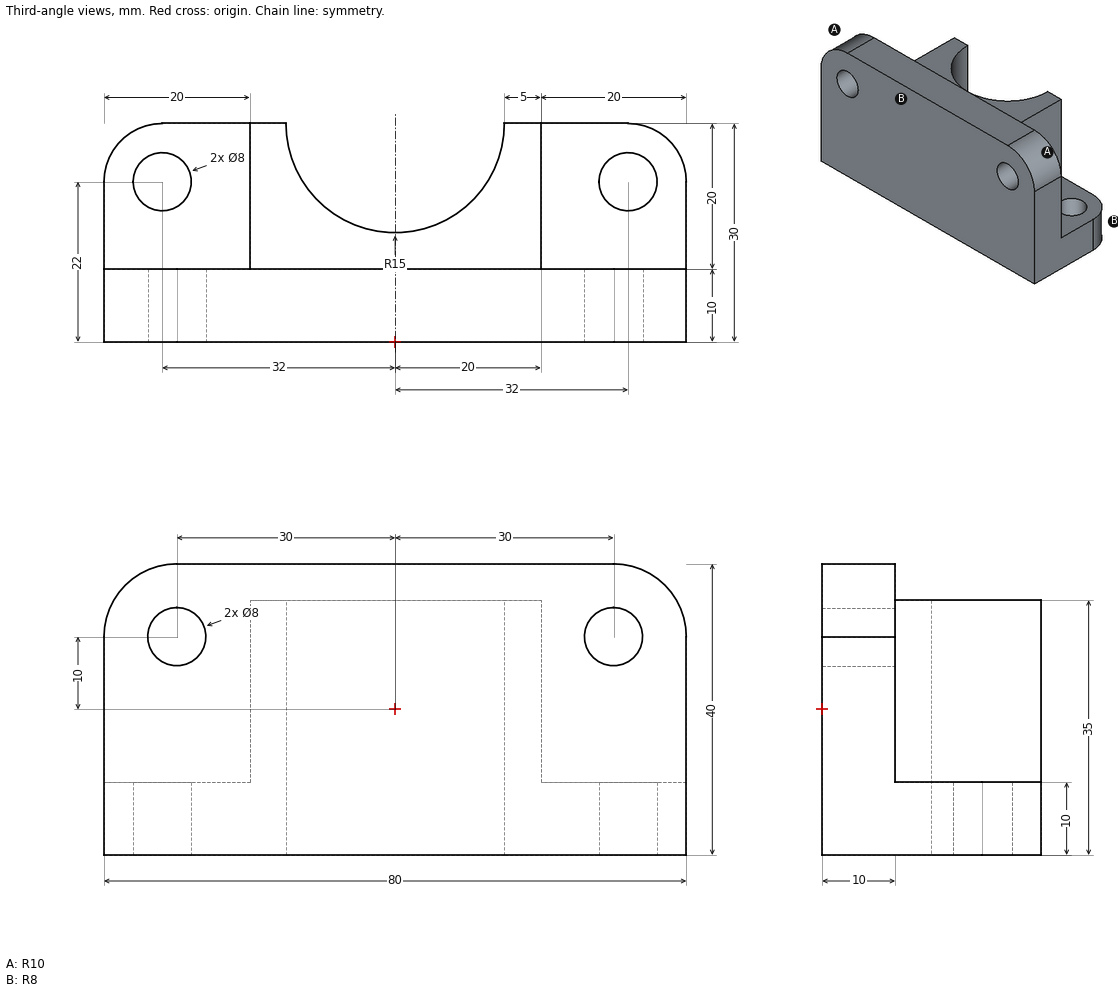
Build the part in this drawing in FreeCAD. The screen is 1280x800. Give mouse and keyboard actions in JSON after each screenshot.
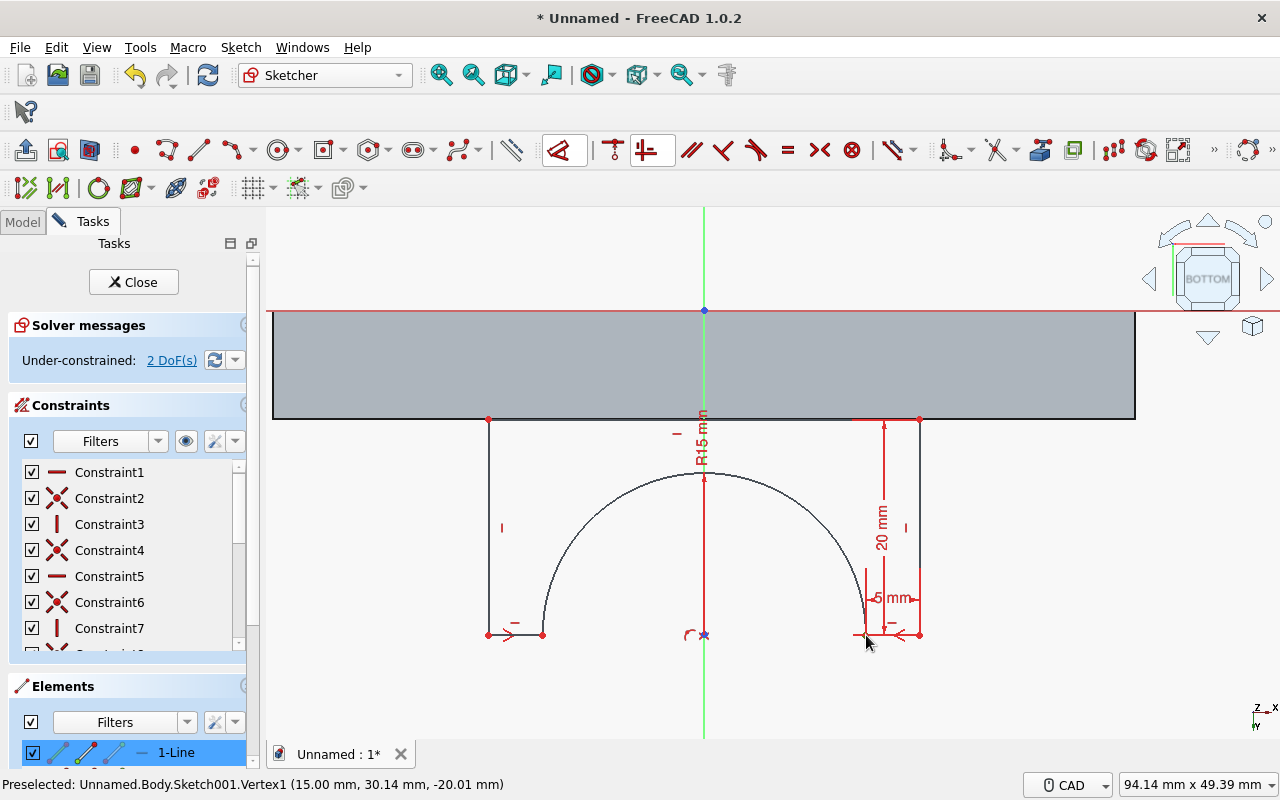
{"action": "key", "text": "i"}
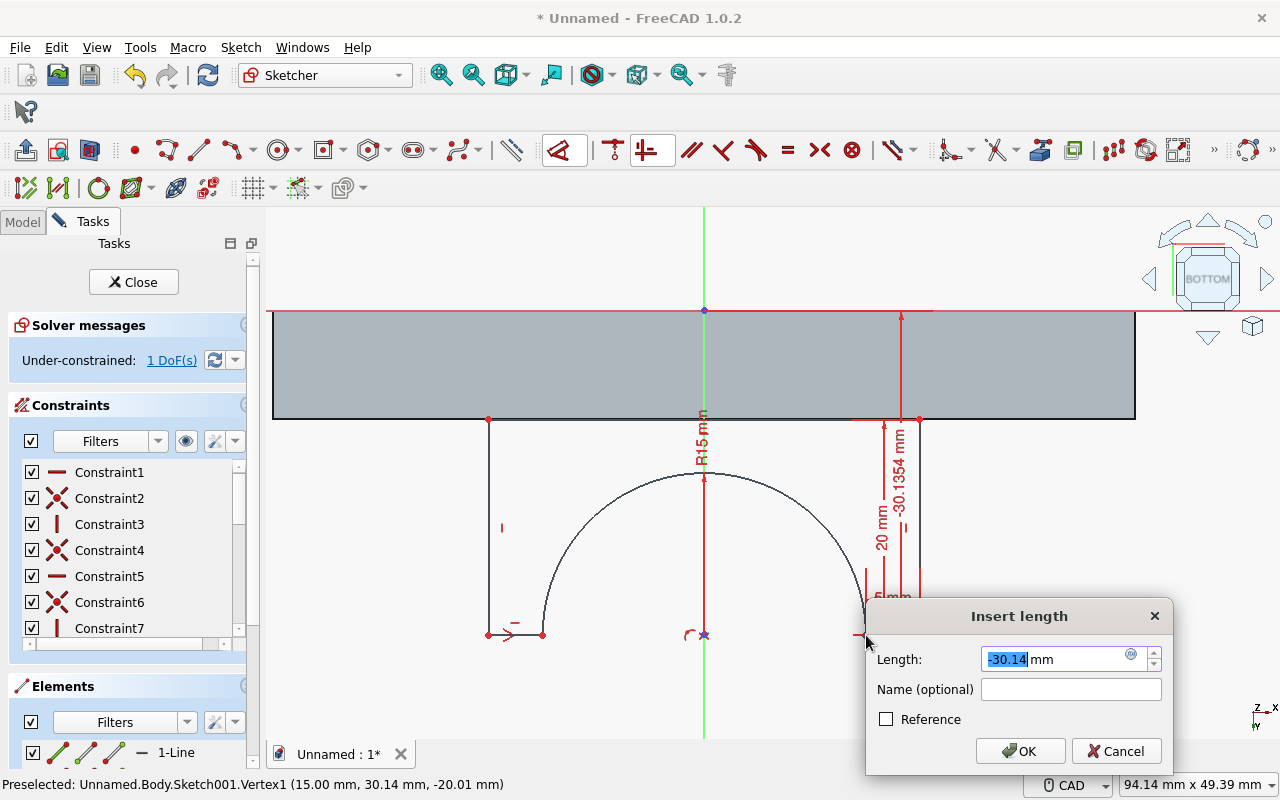
{"action": "type", "text": "-30"}
{"action": "key", "text": "Return"}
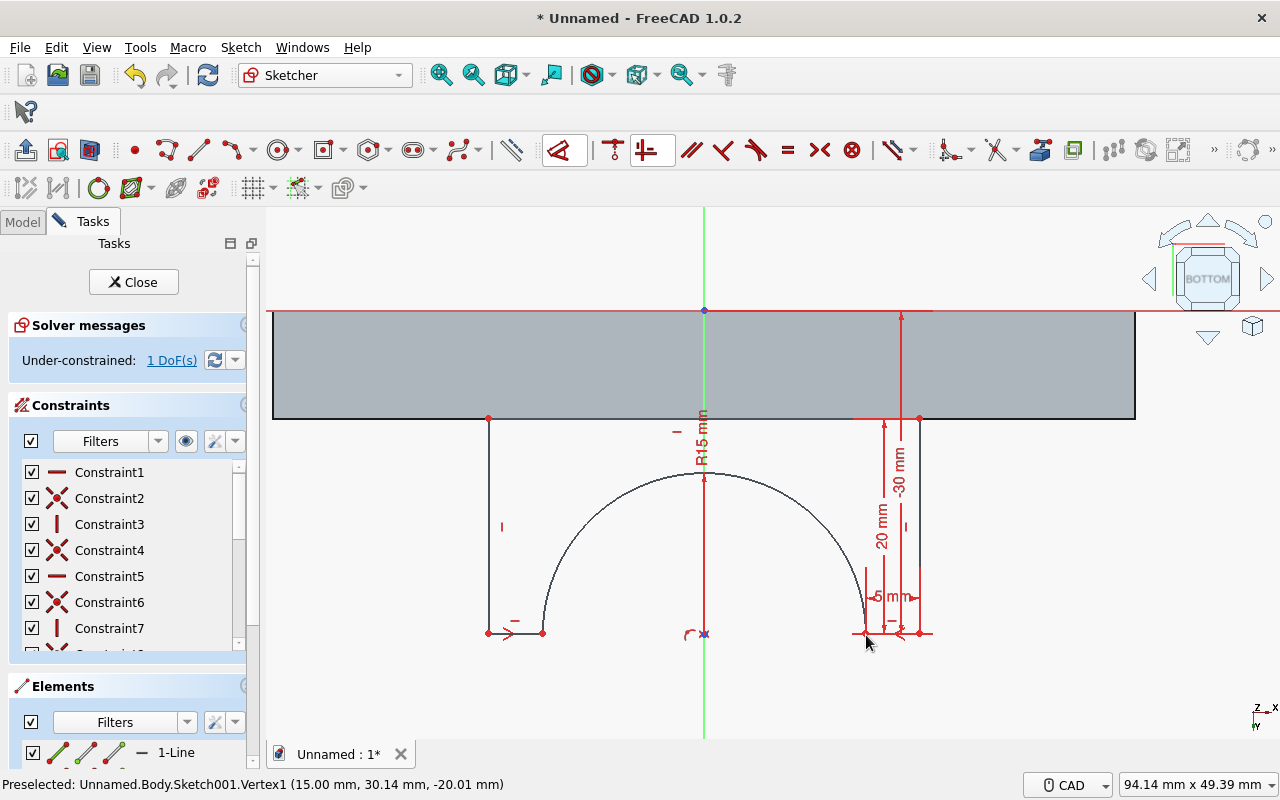
{"action": "left_click", "coordinate": [704, 635]}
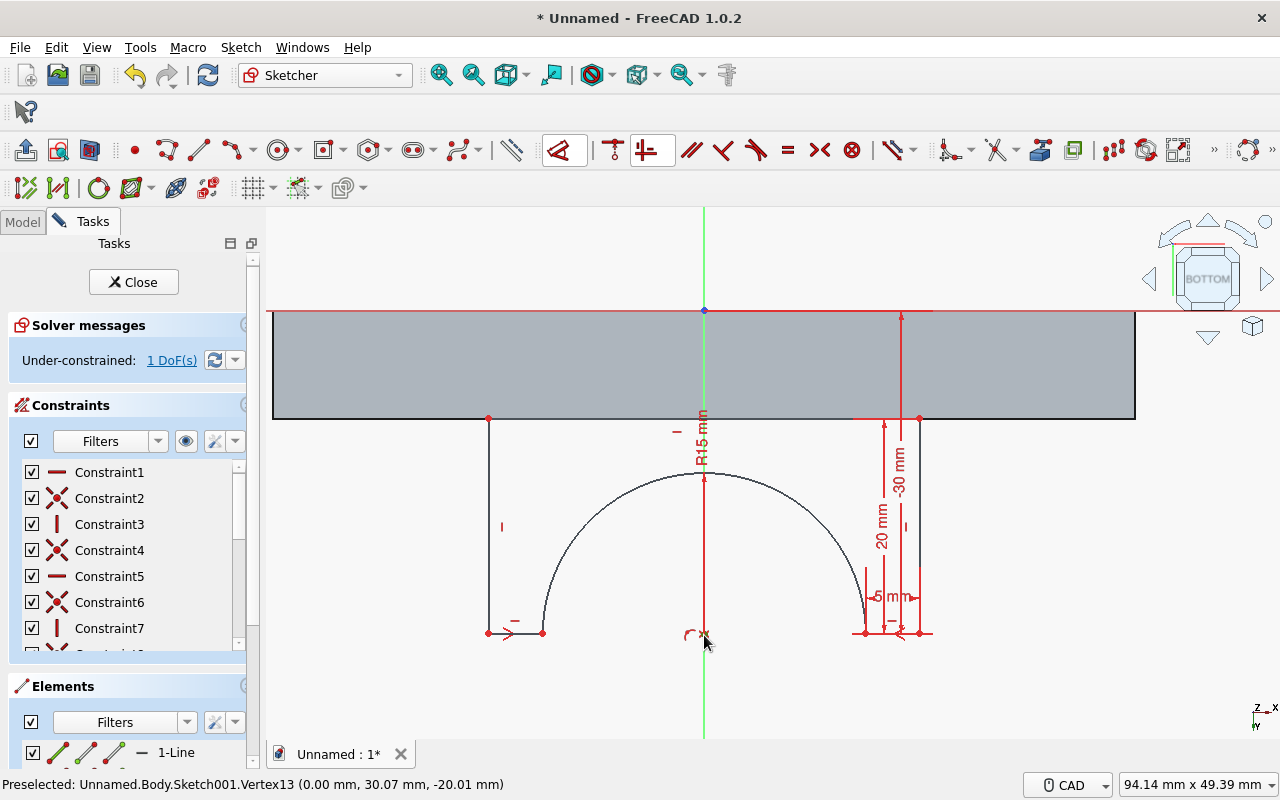
{"action": "left_click", "coordinate": [582, 150]}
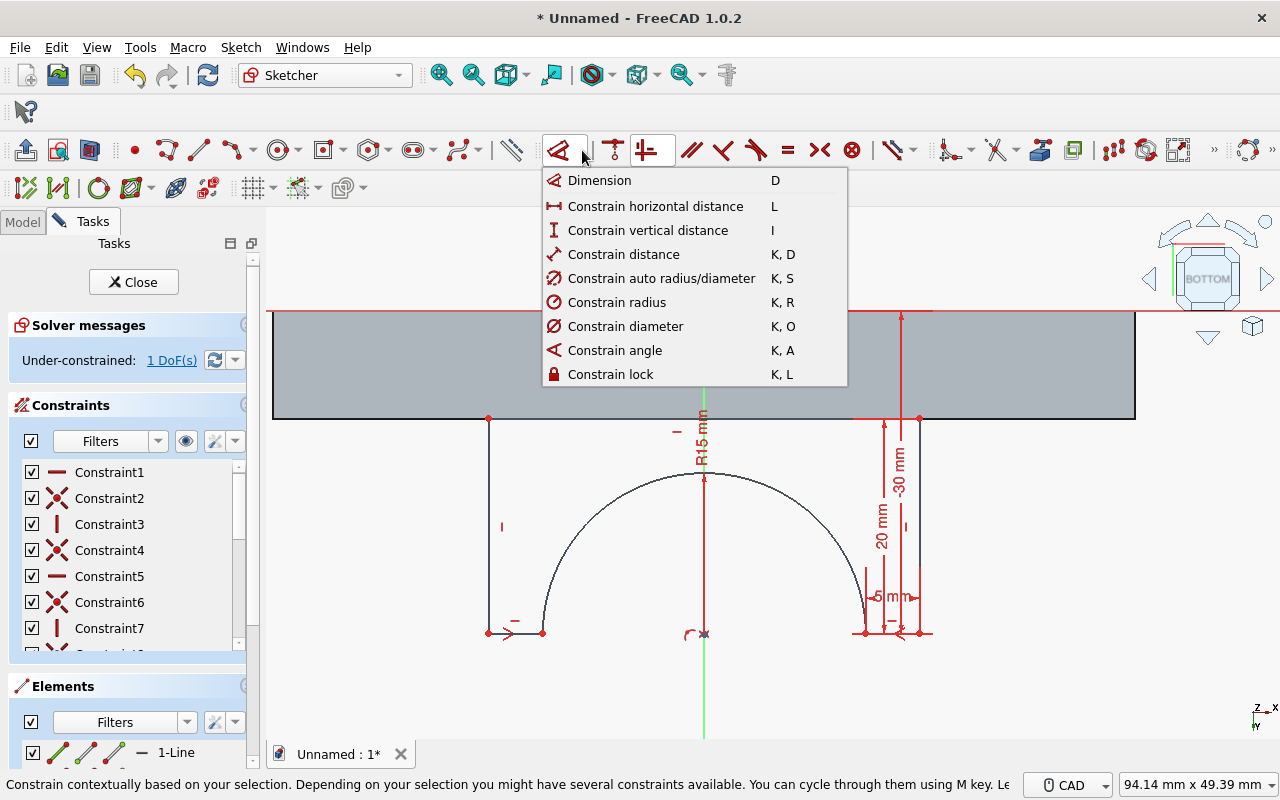
{"action": "left_click", "coordinate": [695, 230]}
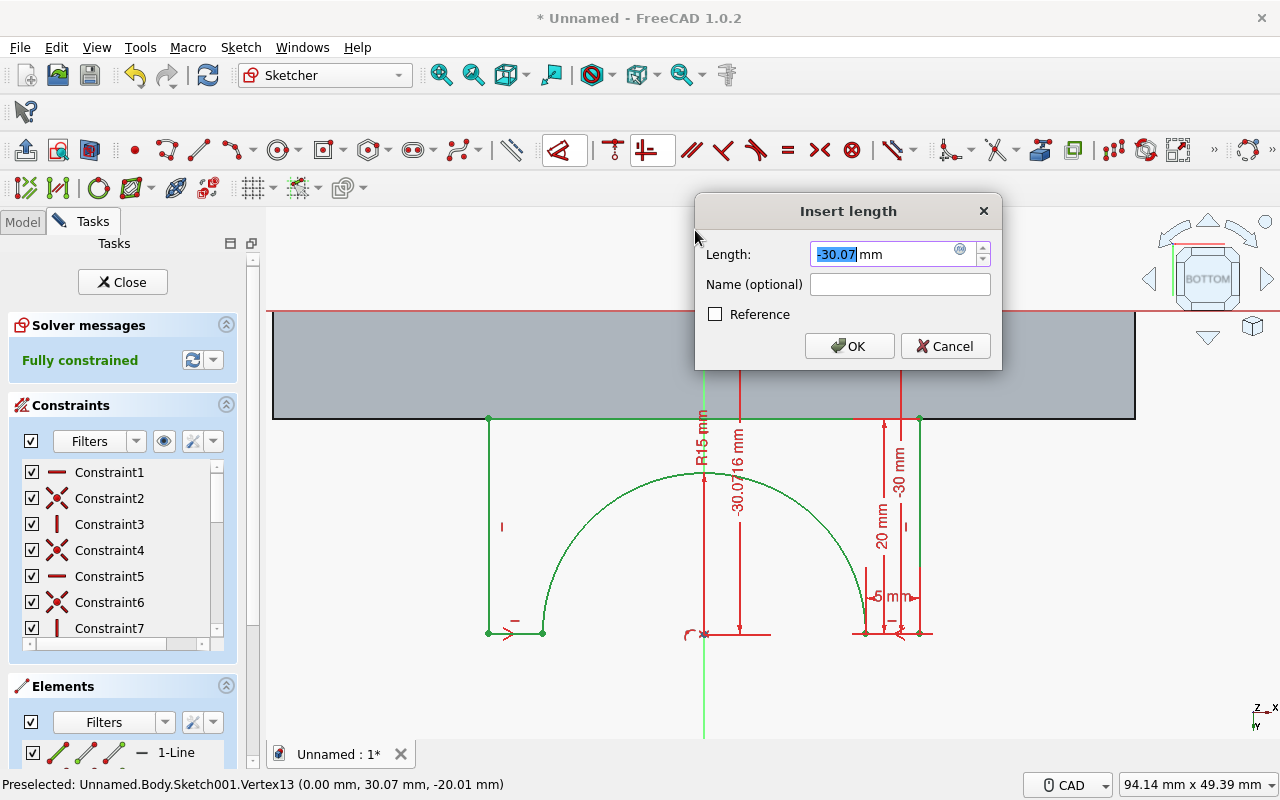
{"action": "type", "text": "-30"}
{"action": "key", "text": "Return"}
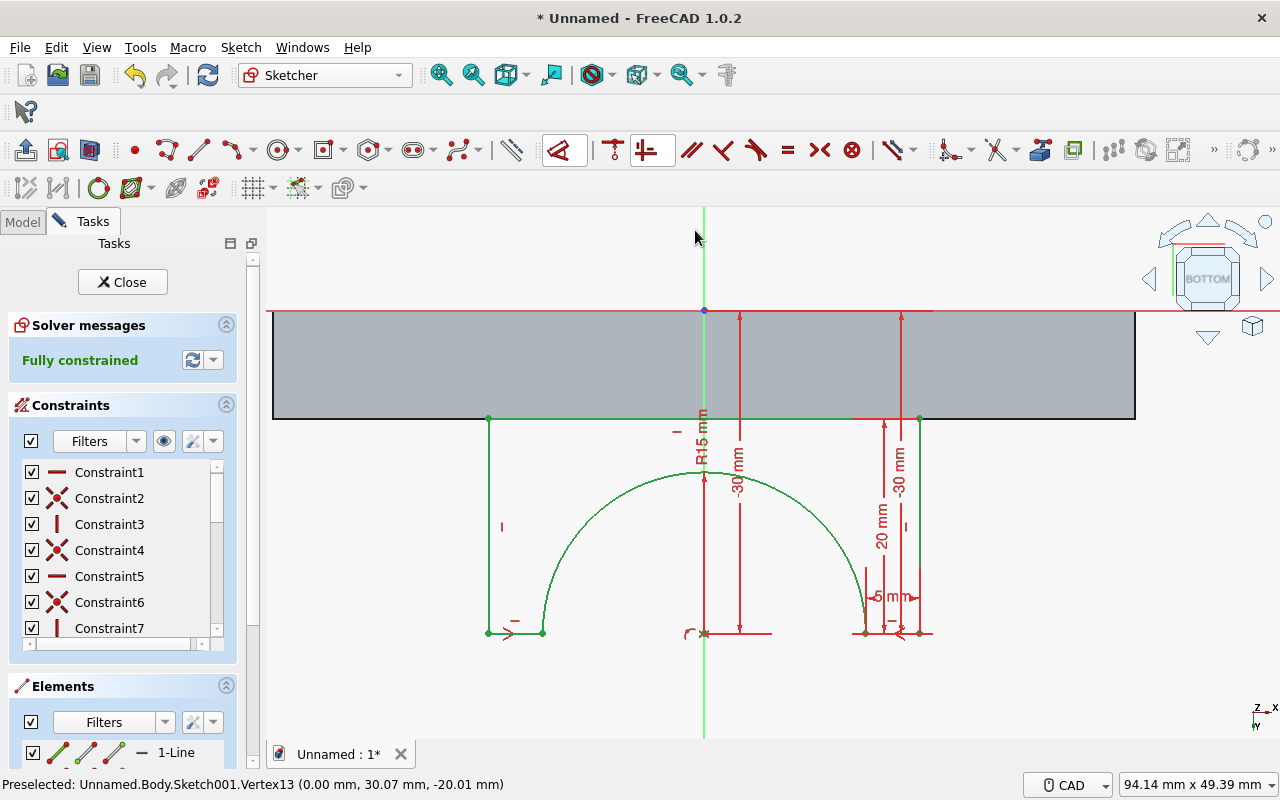
{"action": "left_click", "coordinate": [123, 282]}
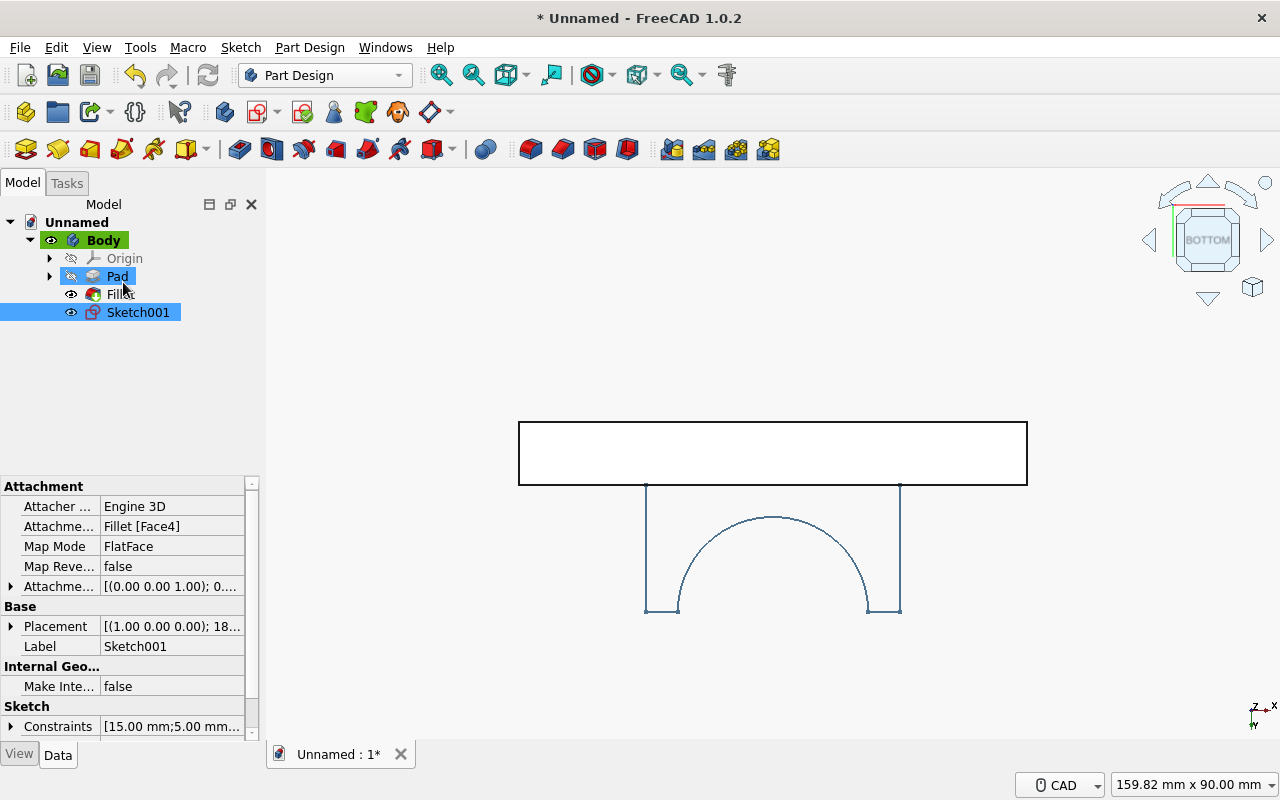
{"action": "left_click", "coordinate": [26, 150]}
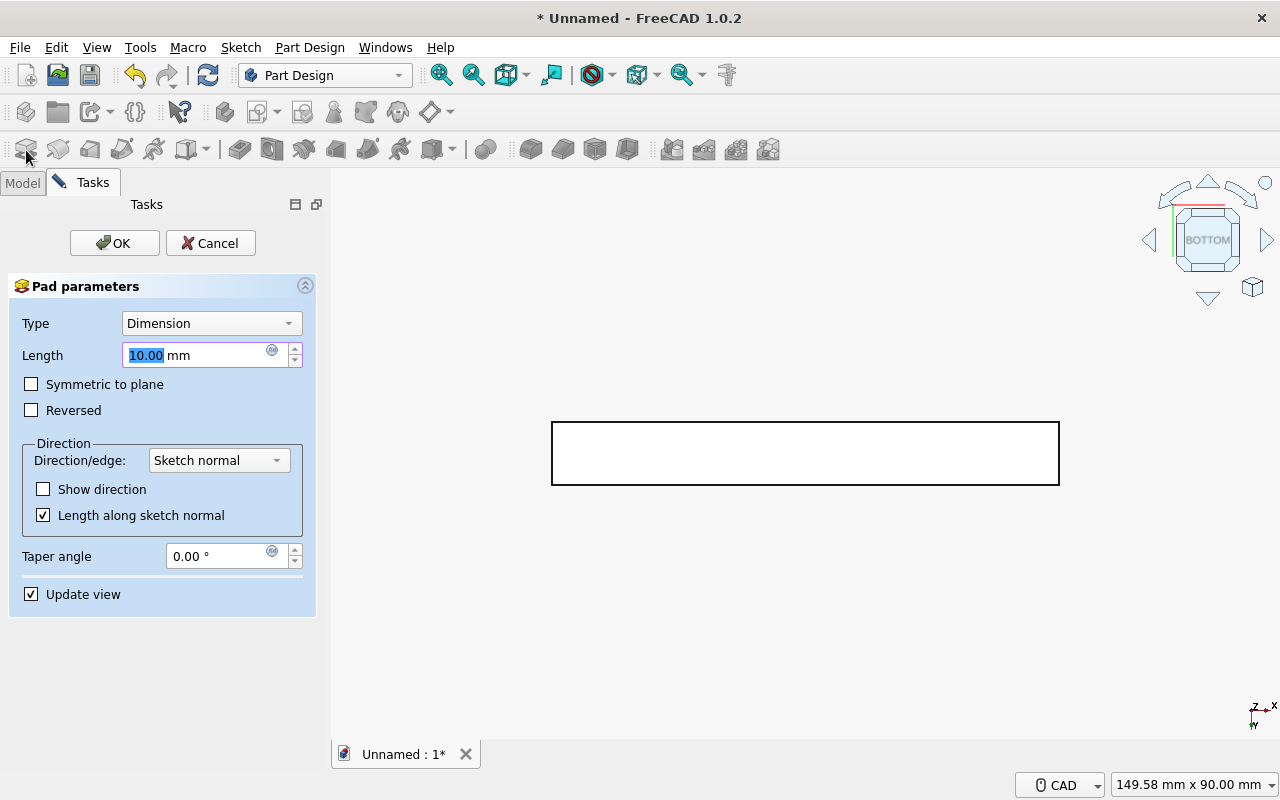
{"action": "type", "text": "35"}
{"action": "key", "text": "Tab"}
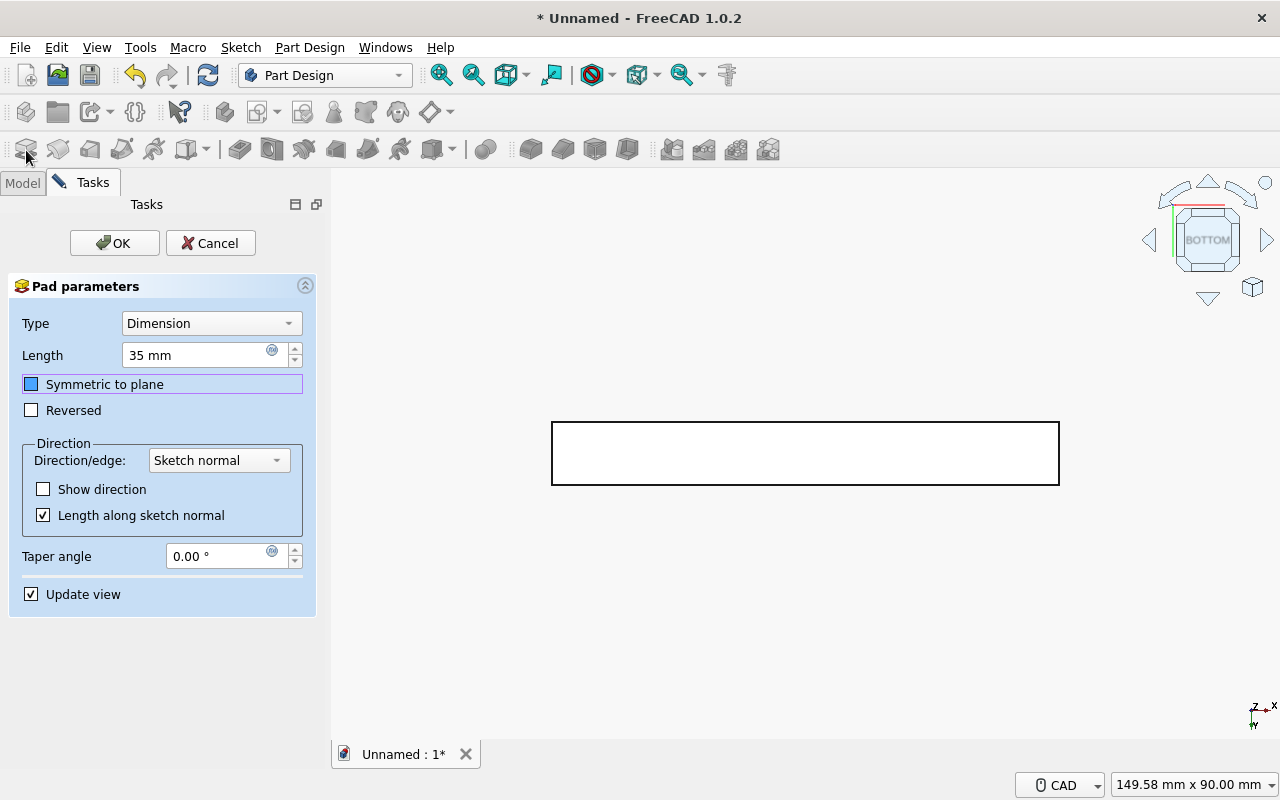
{"action": "left_click", "coordinate": [30, 410]}